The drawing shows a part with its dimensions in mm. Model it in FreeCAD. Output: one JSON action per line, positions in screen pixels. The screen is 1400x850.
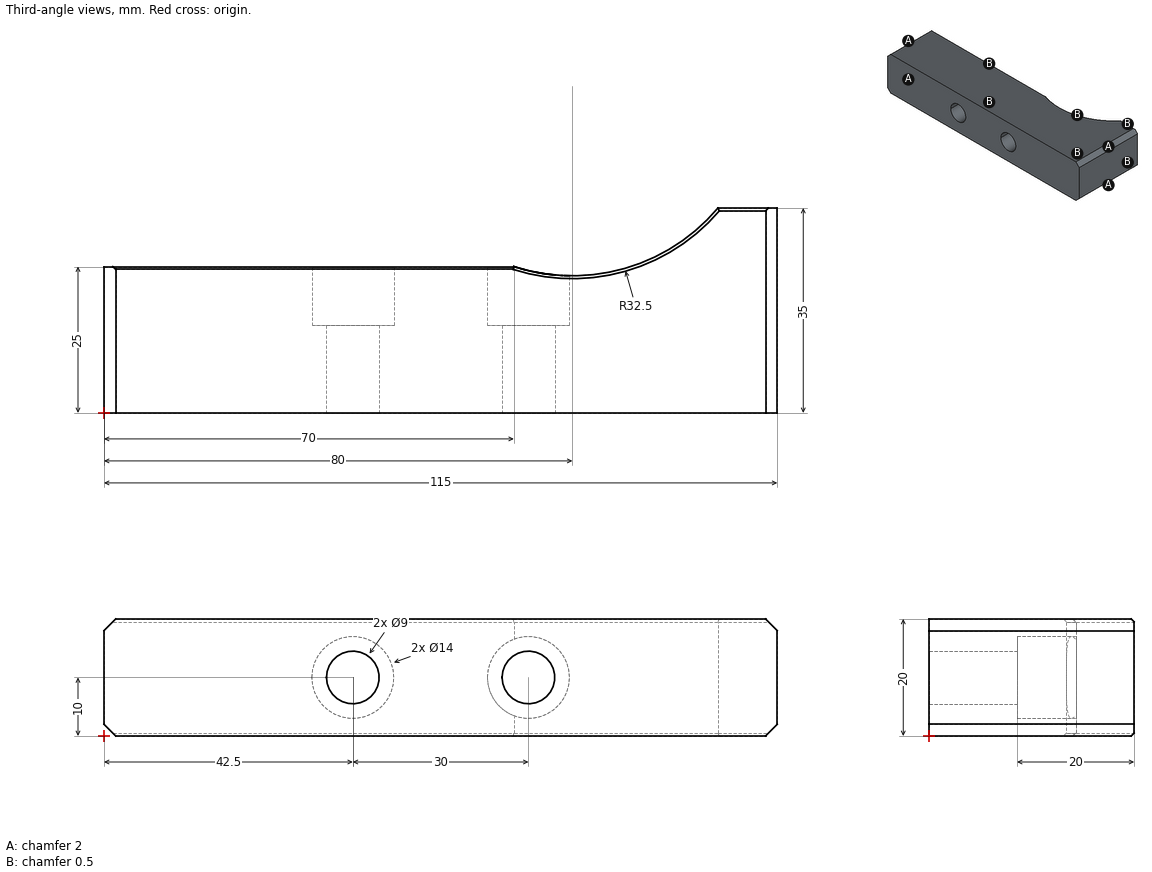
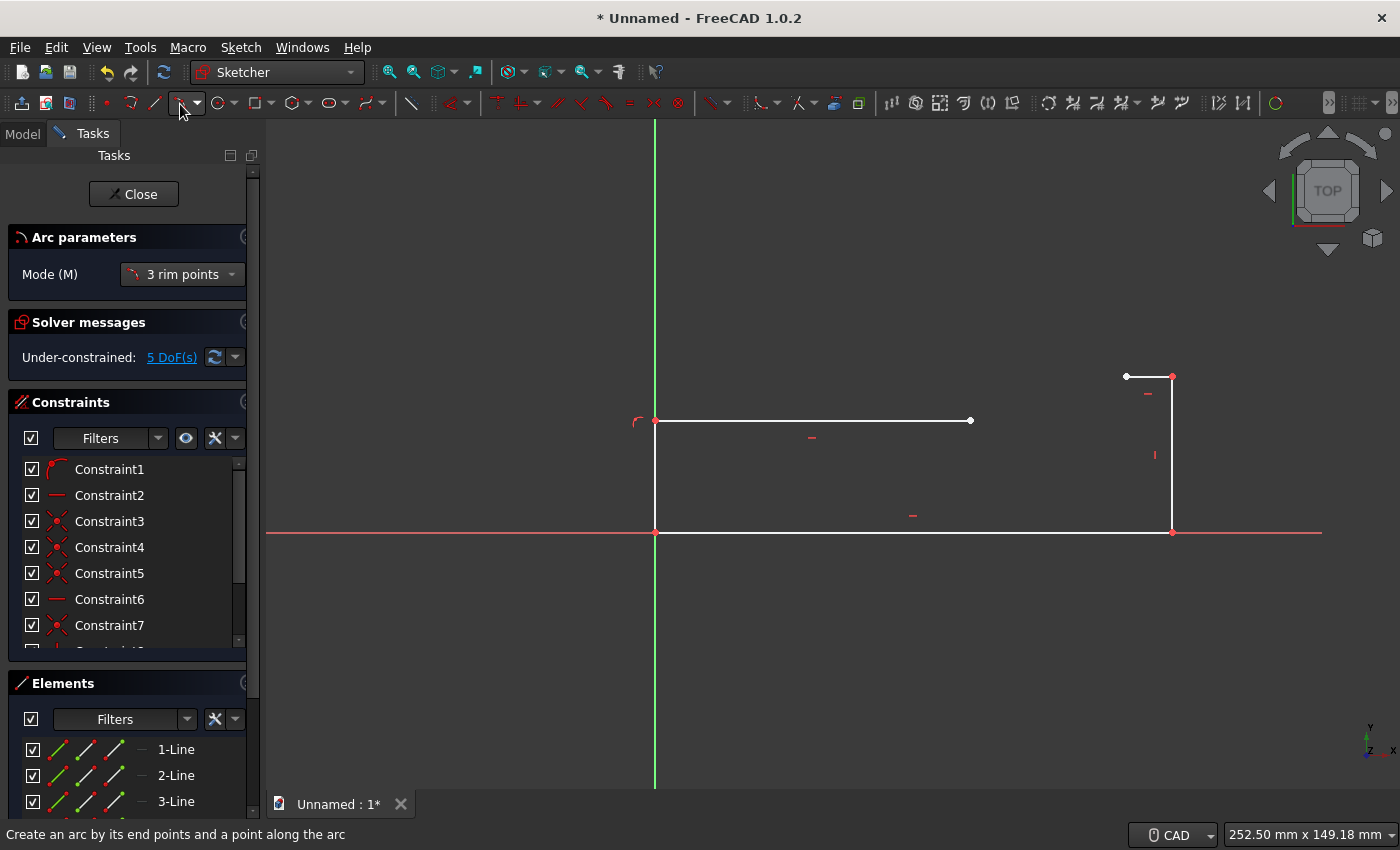
{"action": "left_click", "coordinate": [1126, 377]}
{"action": "left_click", "coordinate": [970, 421]}
{"action": "left_click", "coordinate": [1055, 422]}
{"action": "key", "text": "Escape"}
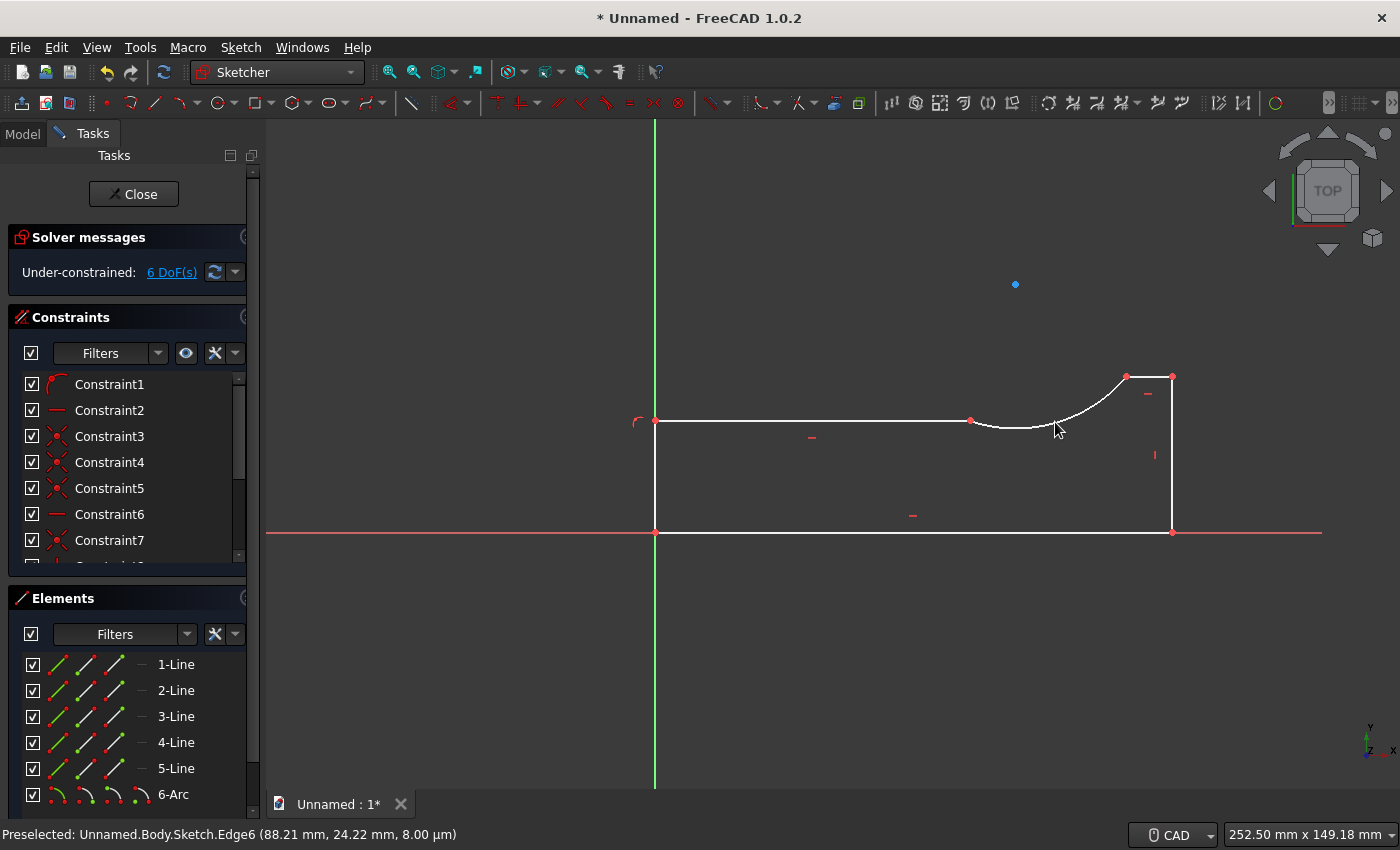
{"action": "left_click", "coordinate": [1021, 428]}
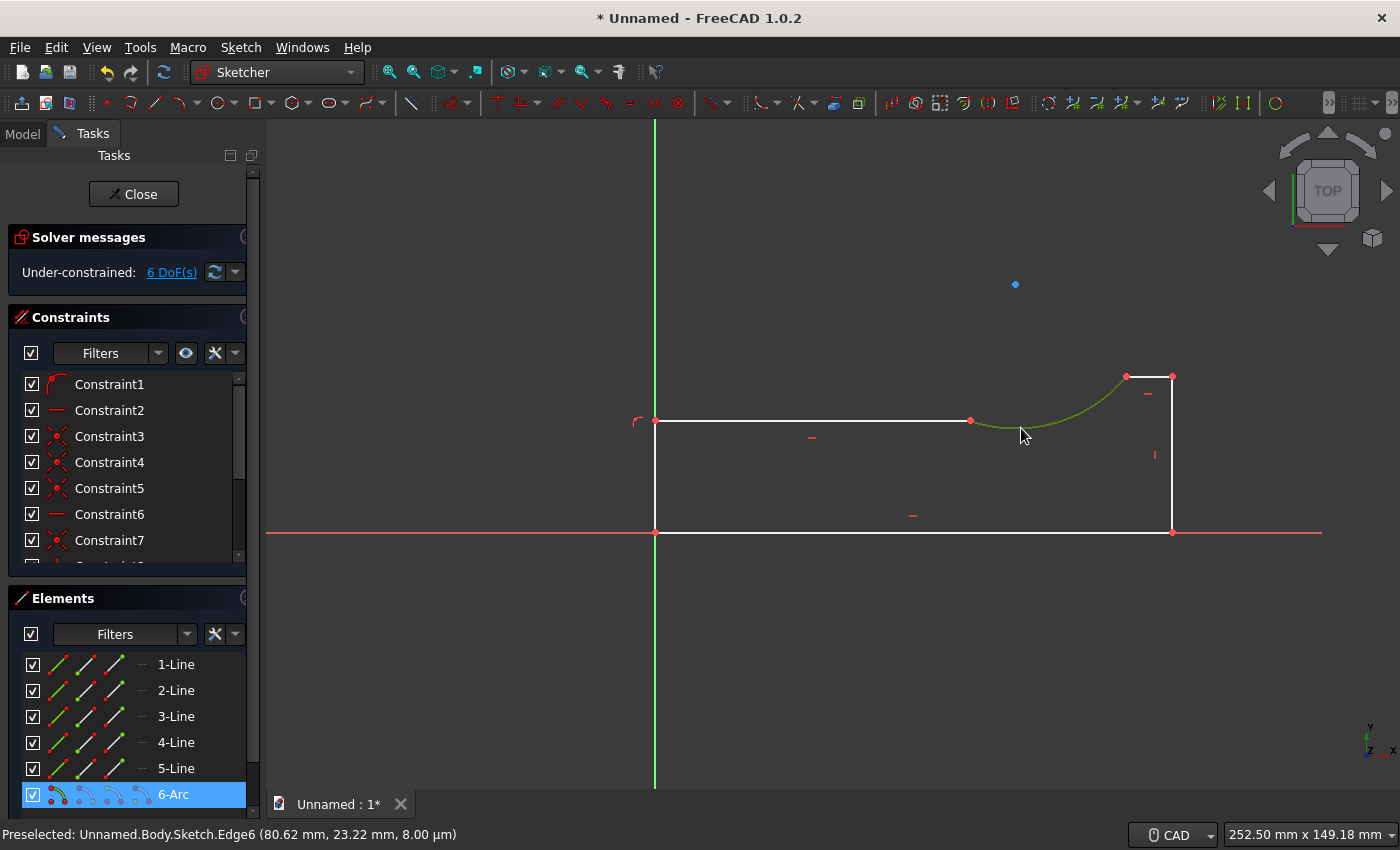
{"action": "left_click", "coordinate": [470, 104]}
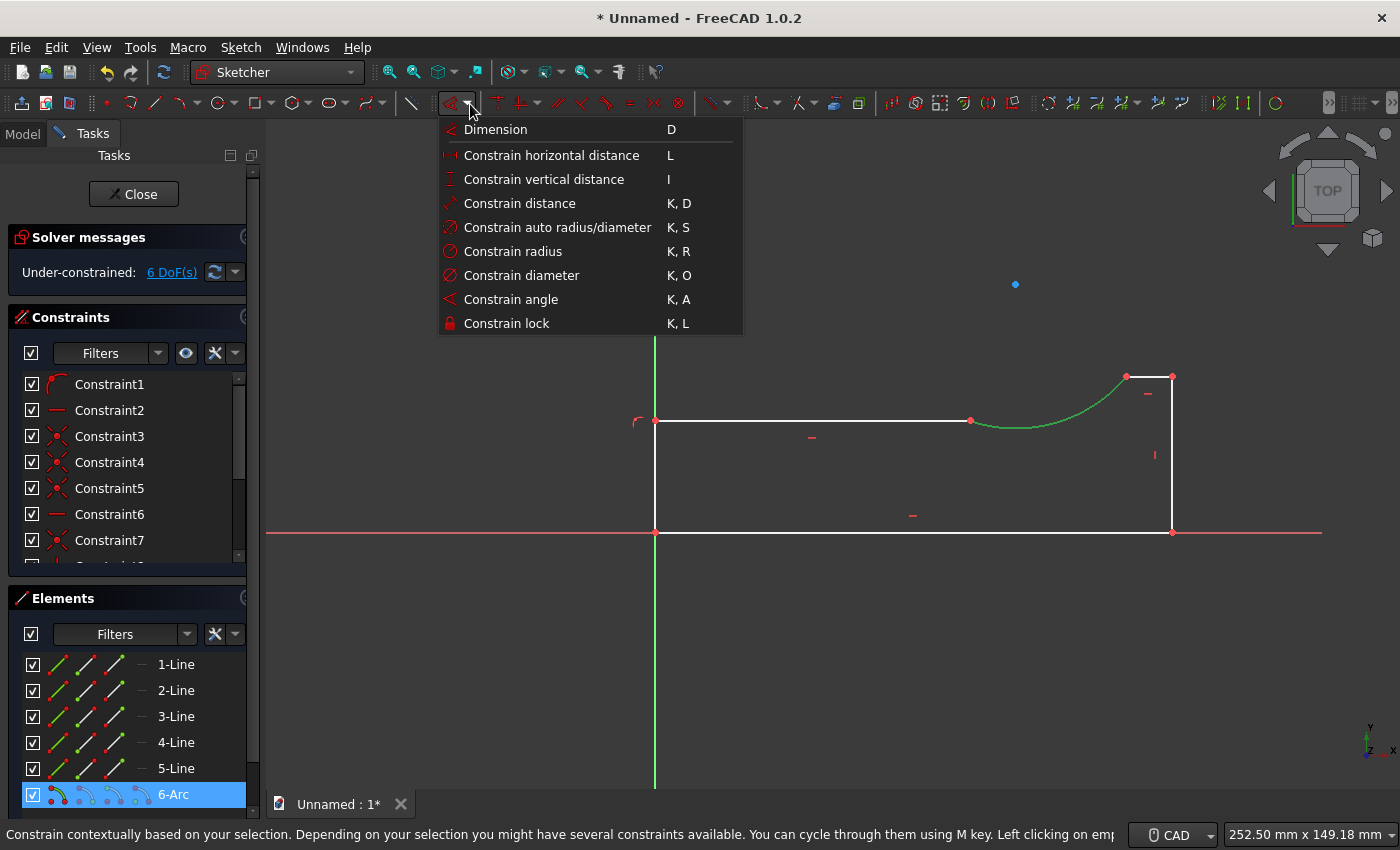
{"action": "left_click", "coordinate": [591, 251]}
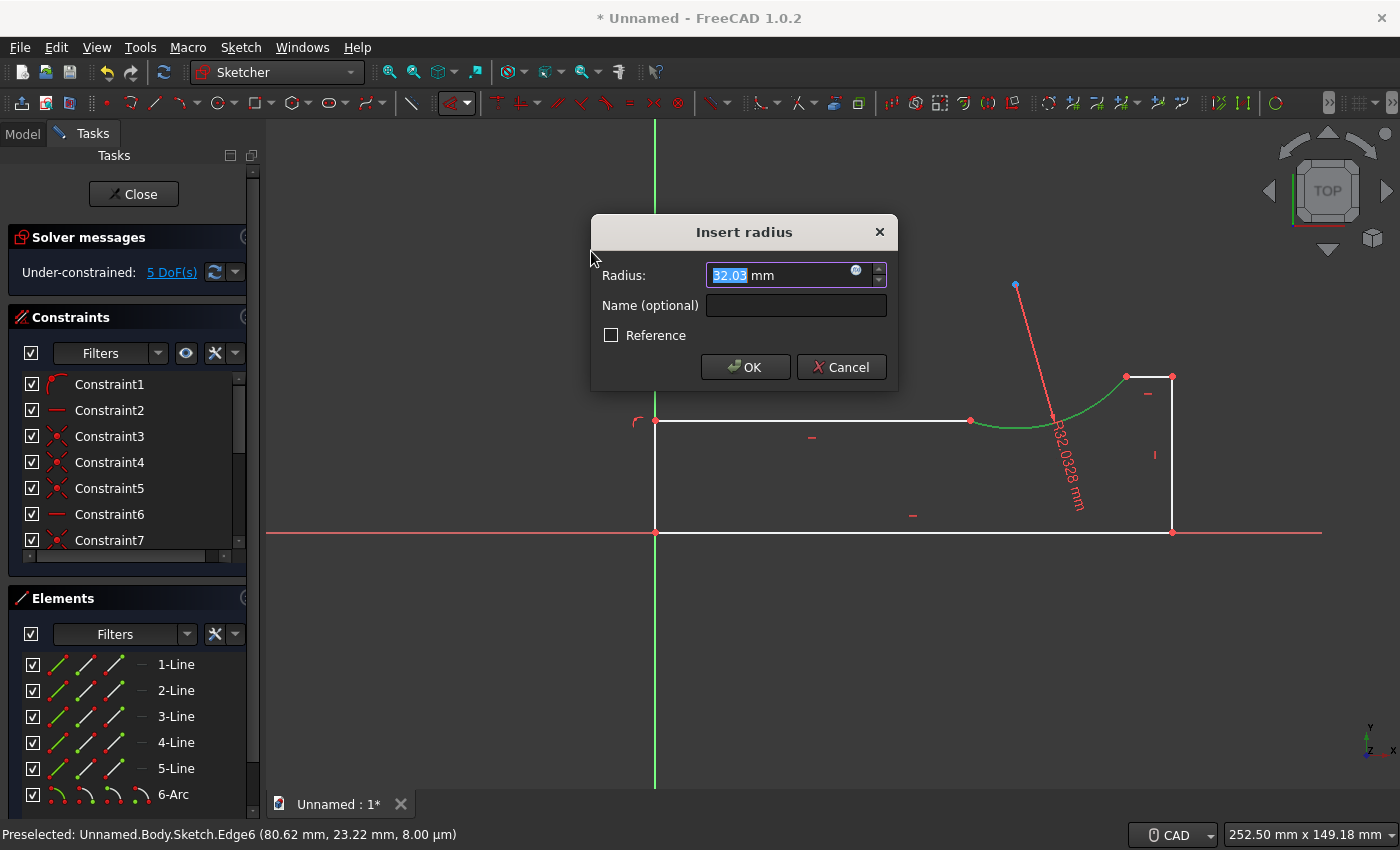
{"action": "type", "text": "32.5"}
{"action": "key", "text": "Return"}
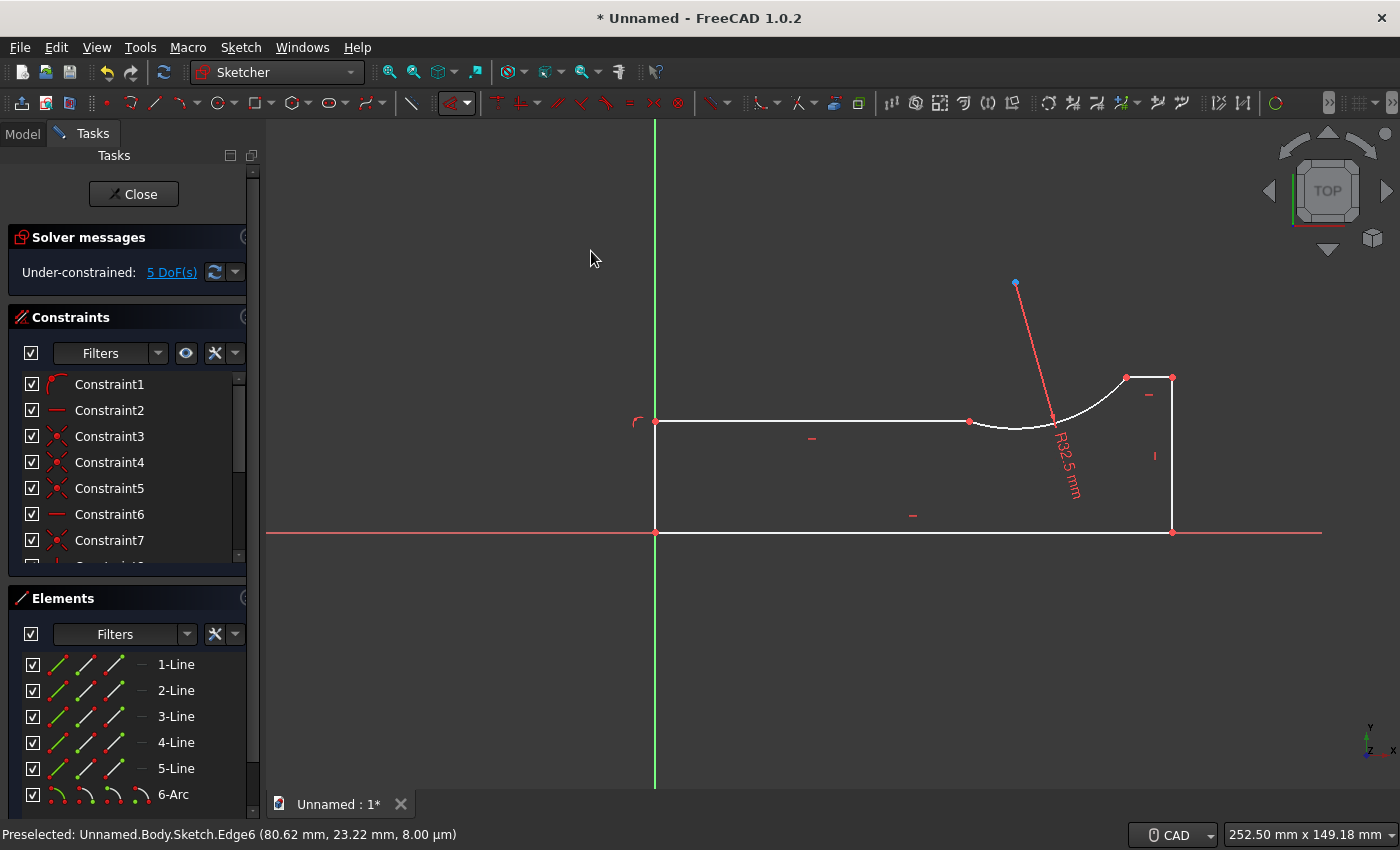
{"action": "left_click", "coordinate": [875, 421]}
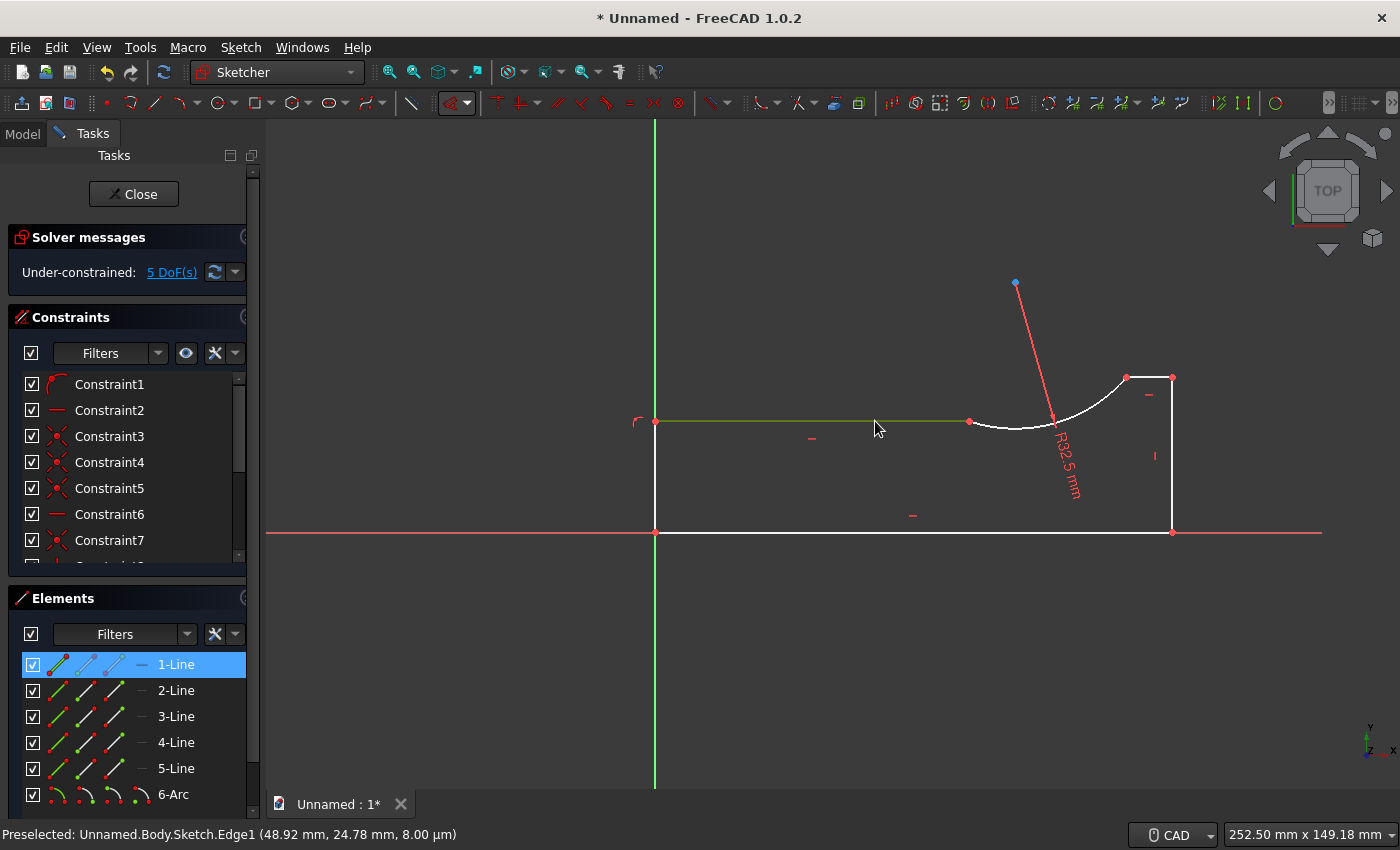
{"action": "left_click", "coordinate": [470, 104]}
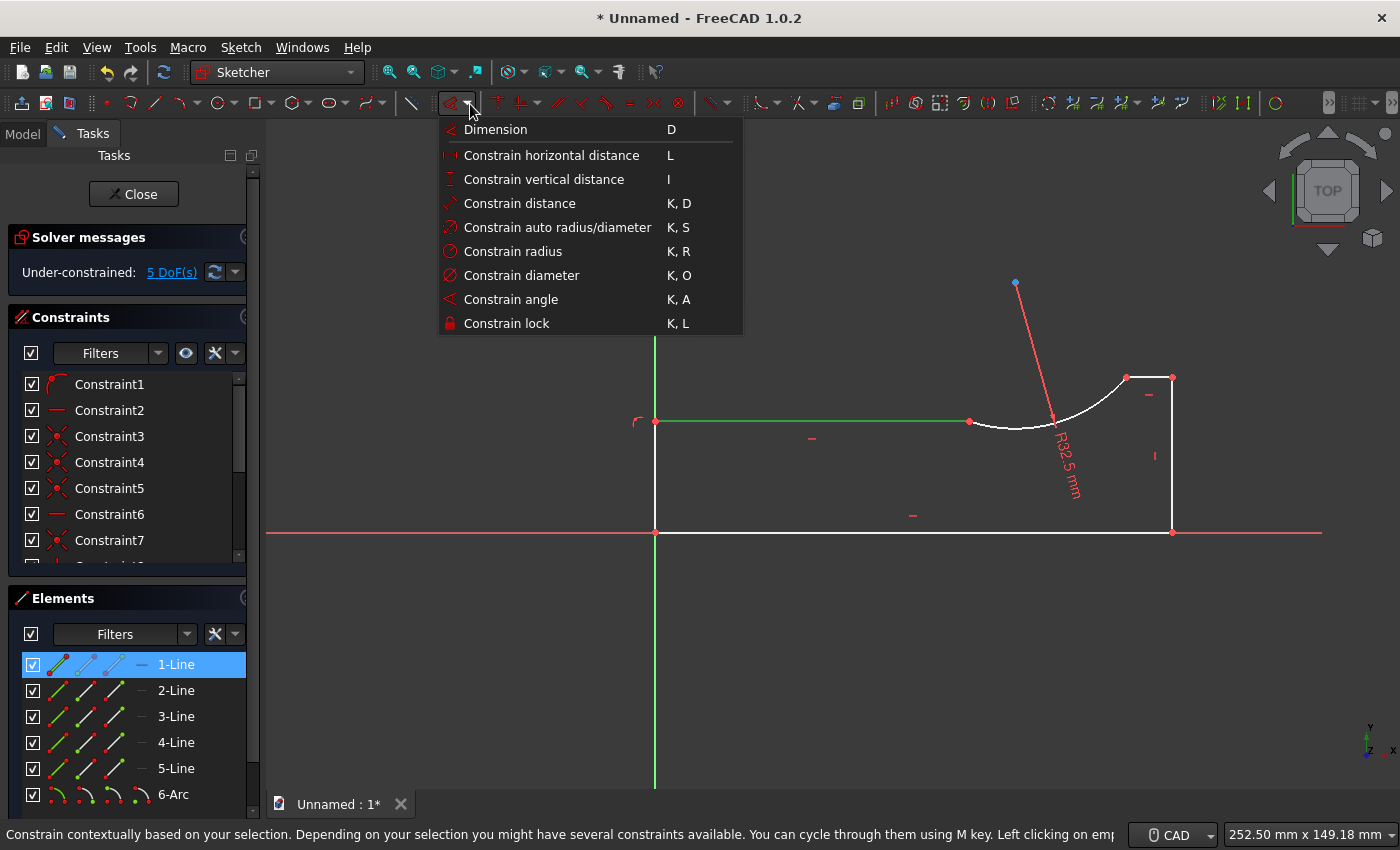
{"action": "left_click", "coordinate": [591, 155]}